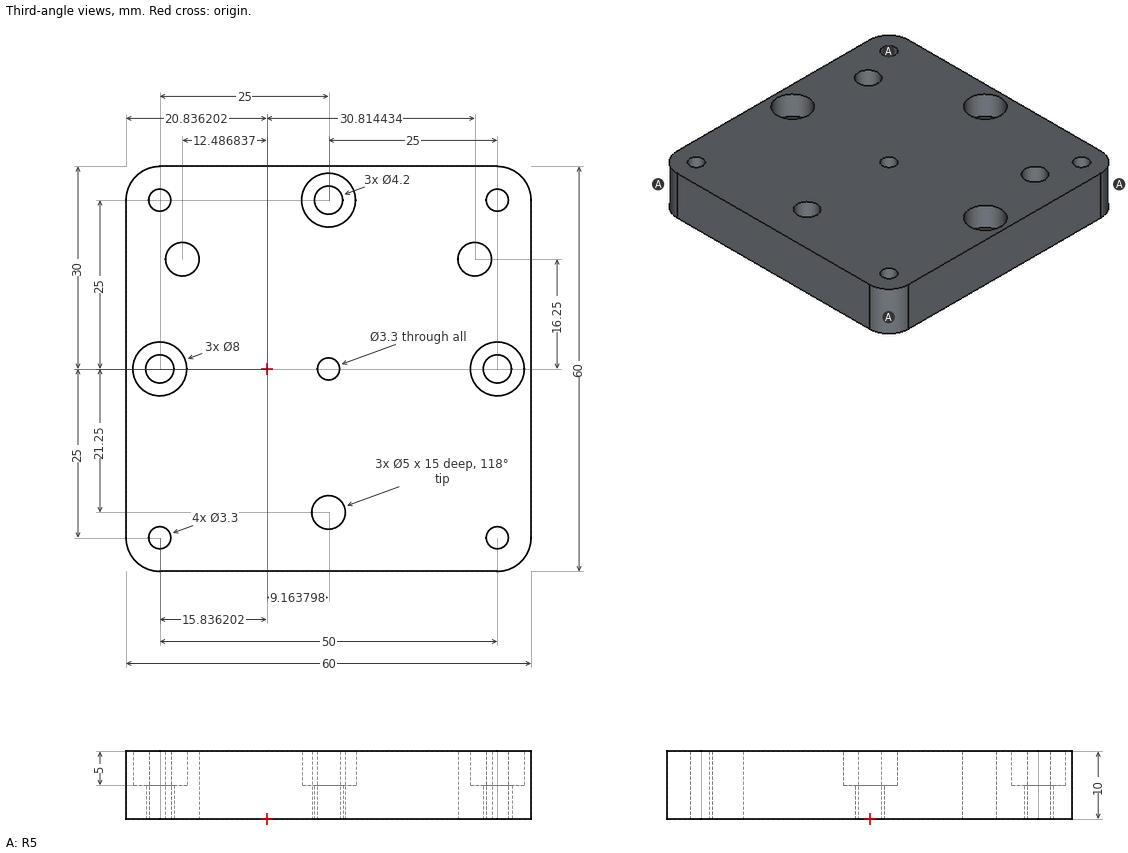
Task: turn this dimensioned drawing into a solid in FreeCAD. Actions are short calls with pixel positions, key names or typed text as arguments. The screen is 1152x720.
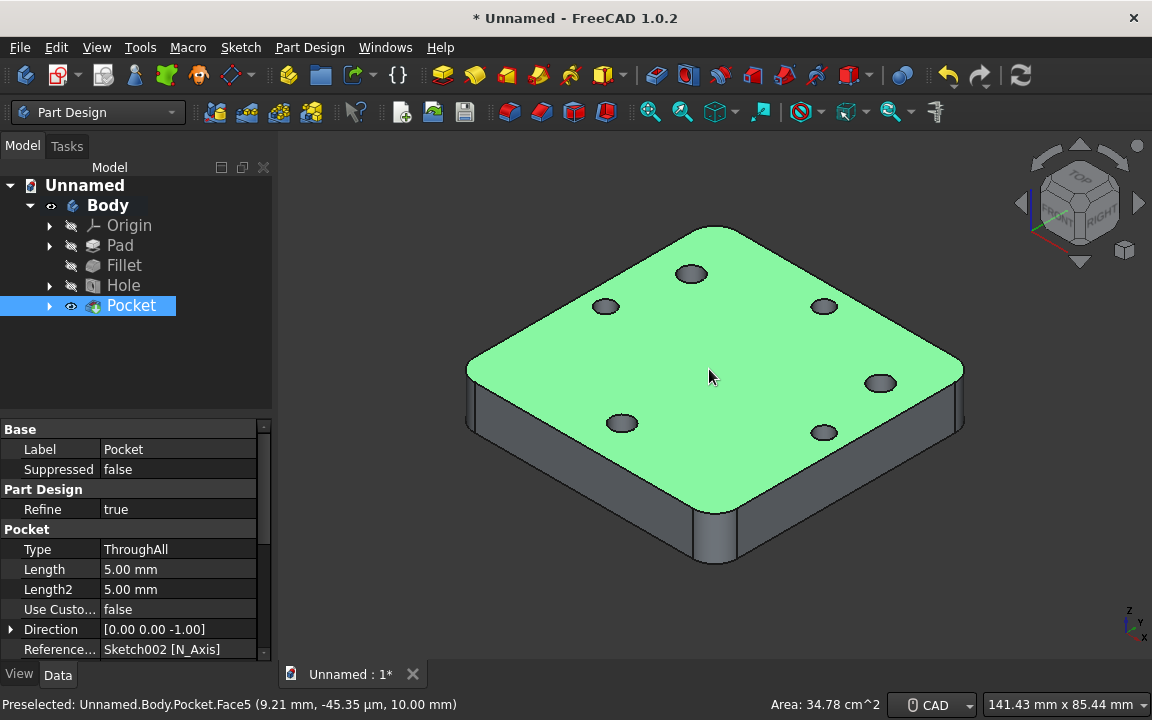
click(58, 76)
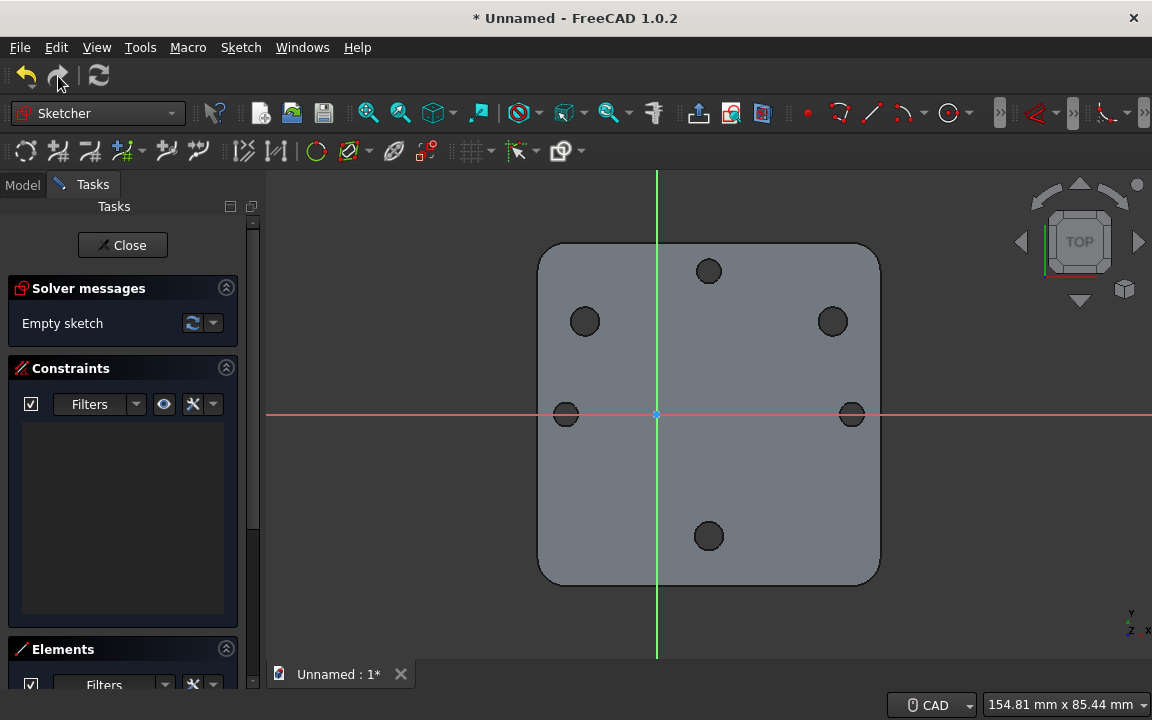
scroll(848, 198, up, 2)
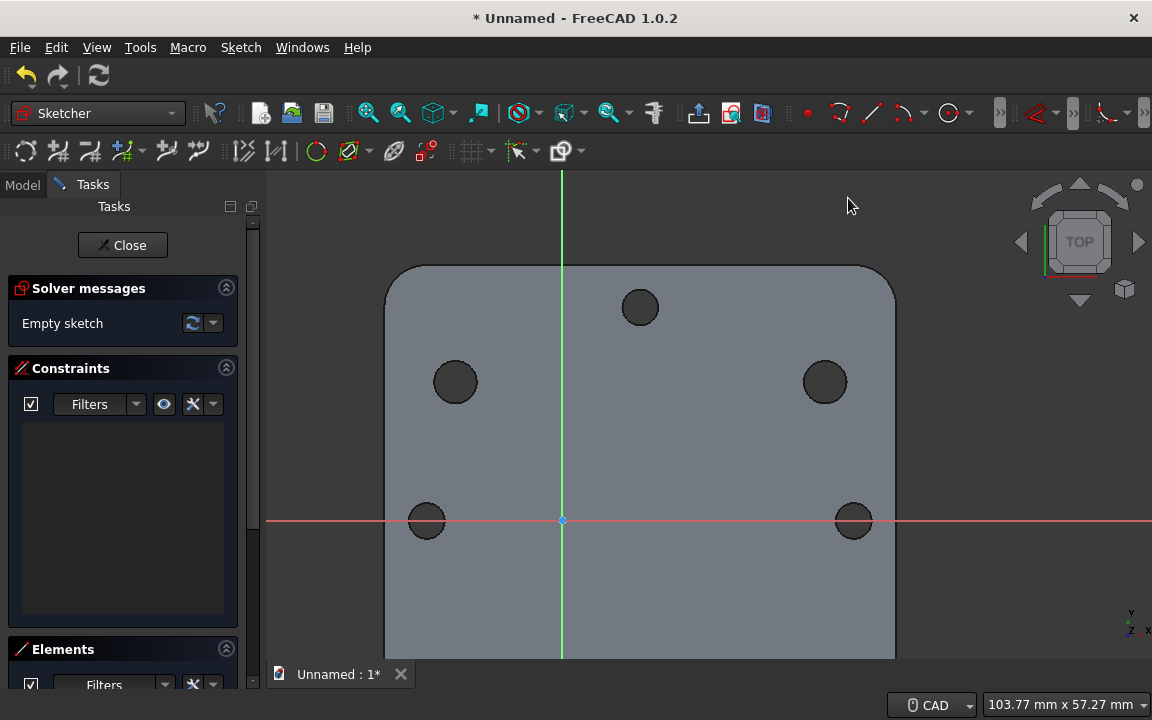
click(950, 114)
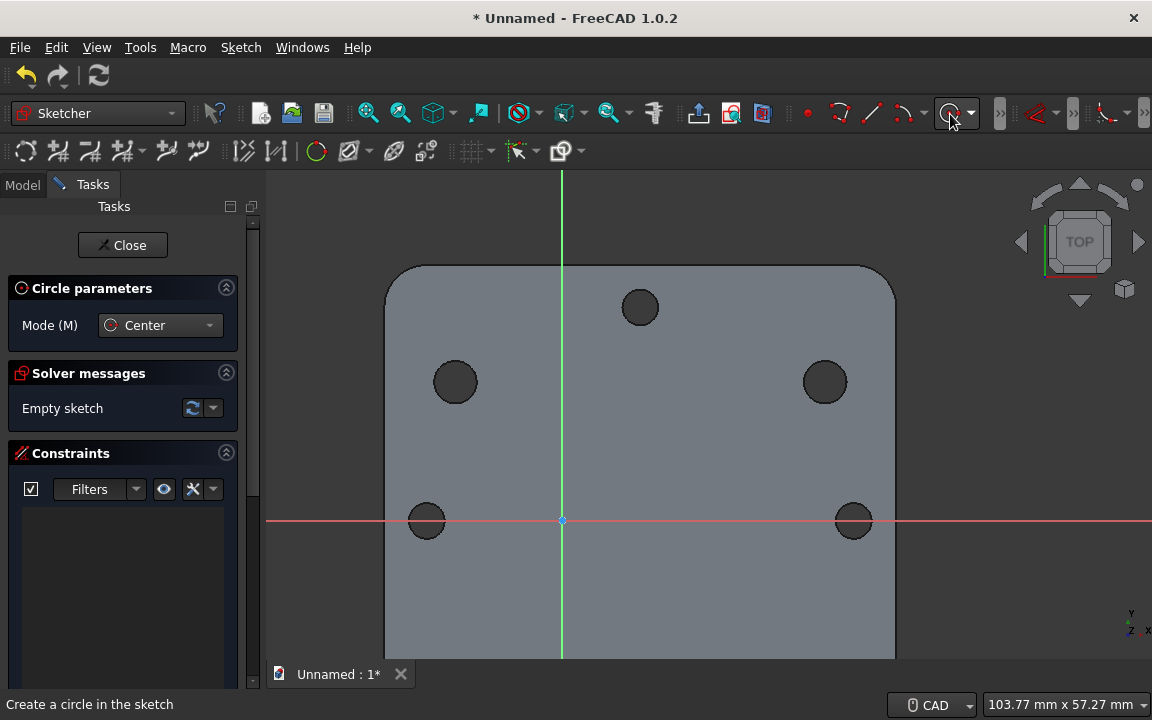
click(427, 521)
move(451, 497)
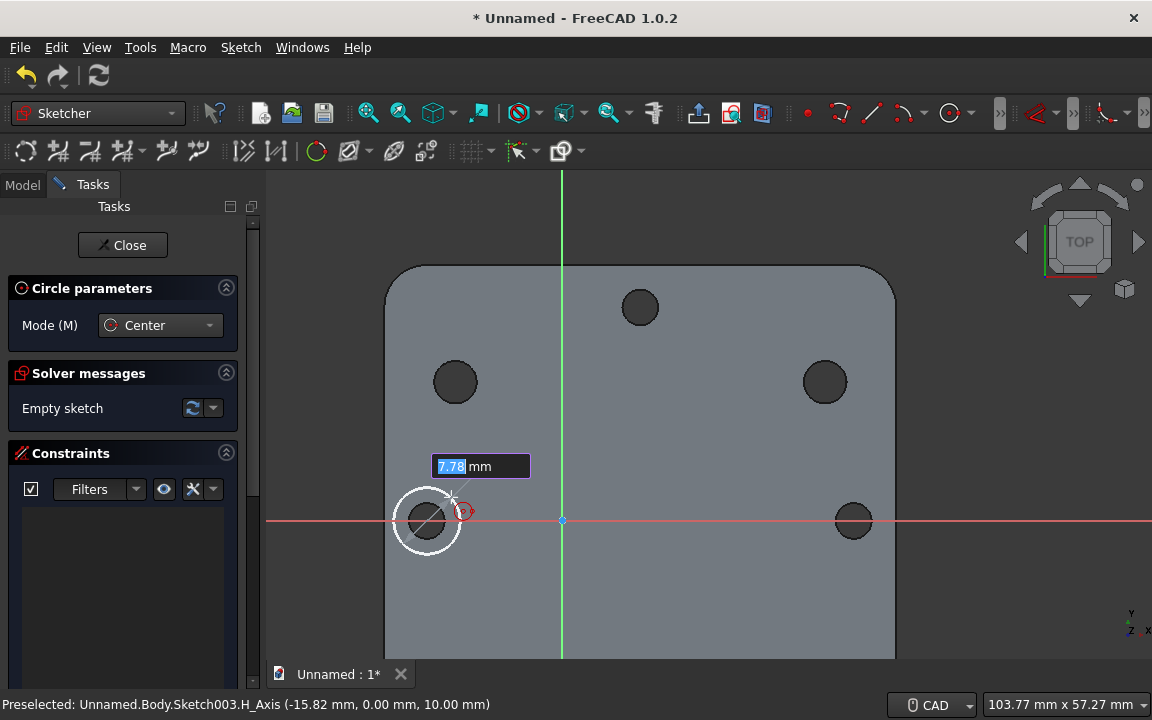
text(8)
key(Return)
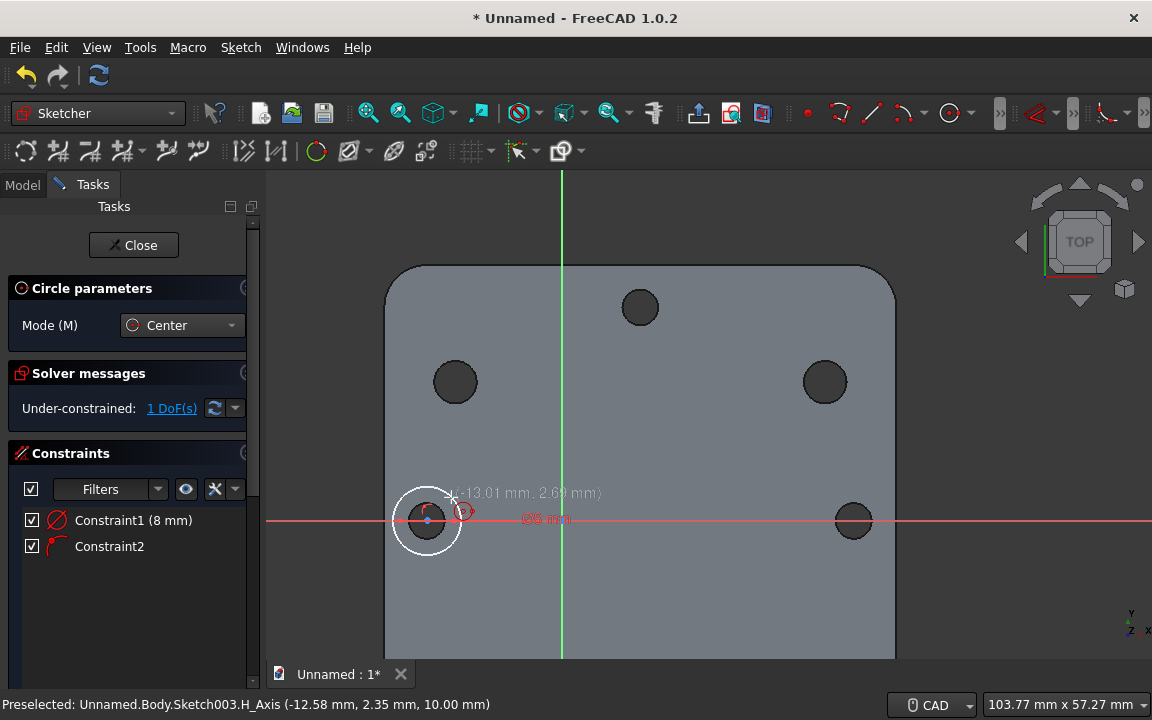
click(640, 307)
move(664, 283)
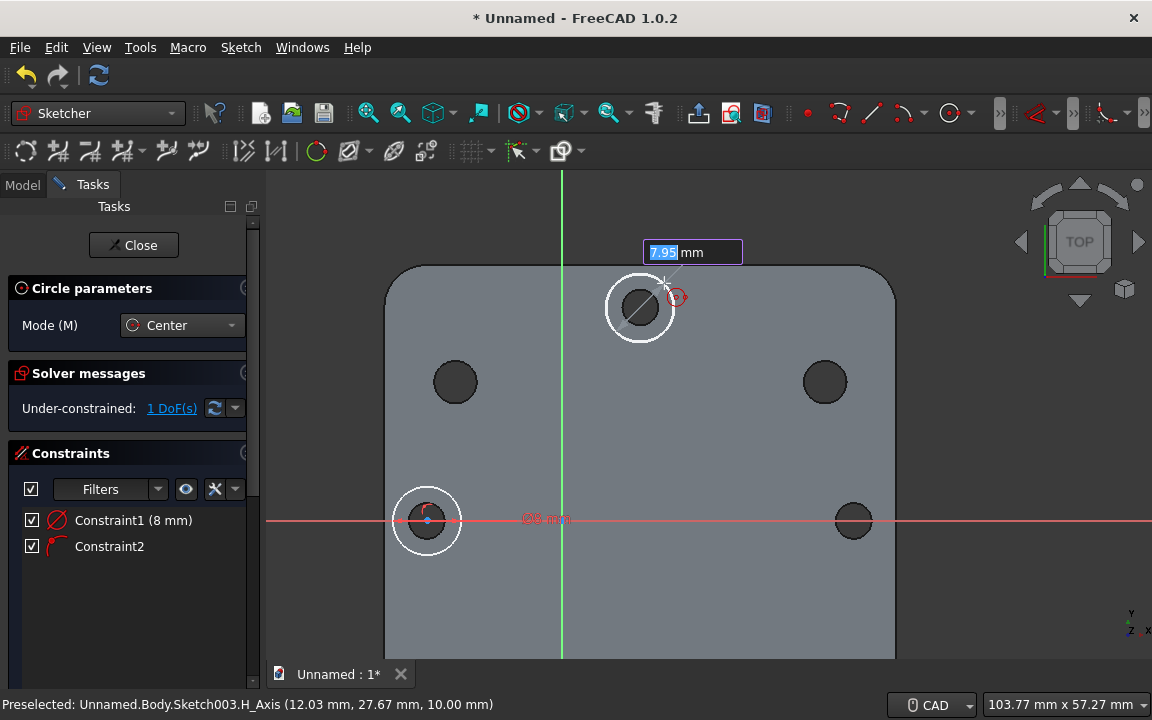
text(8)
key(Return)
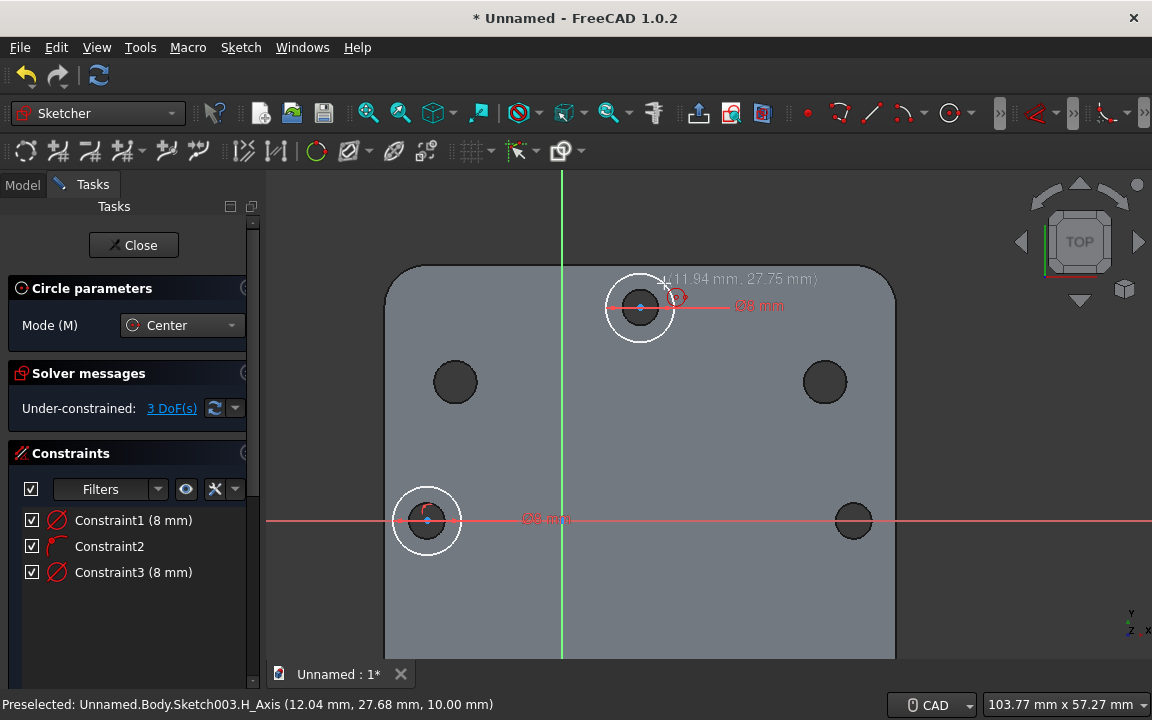
click(854, 521)
move(878, 497)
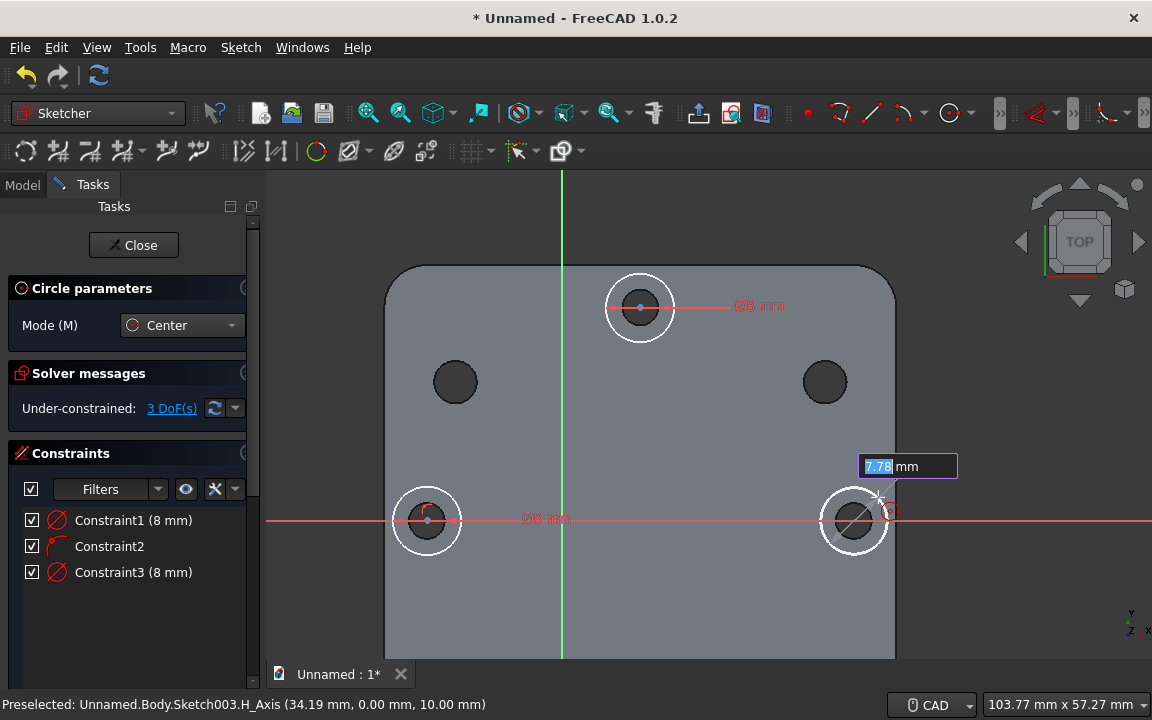
text(8)
key(Return)
key(Escape)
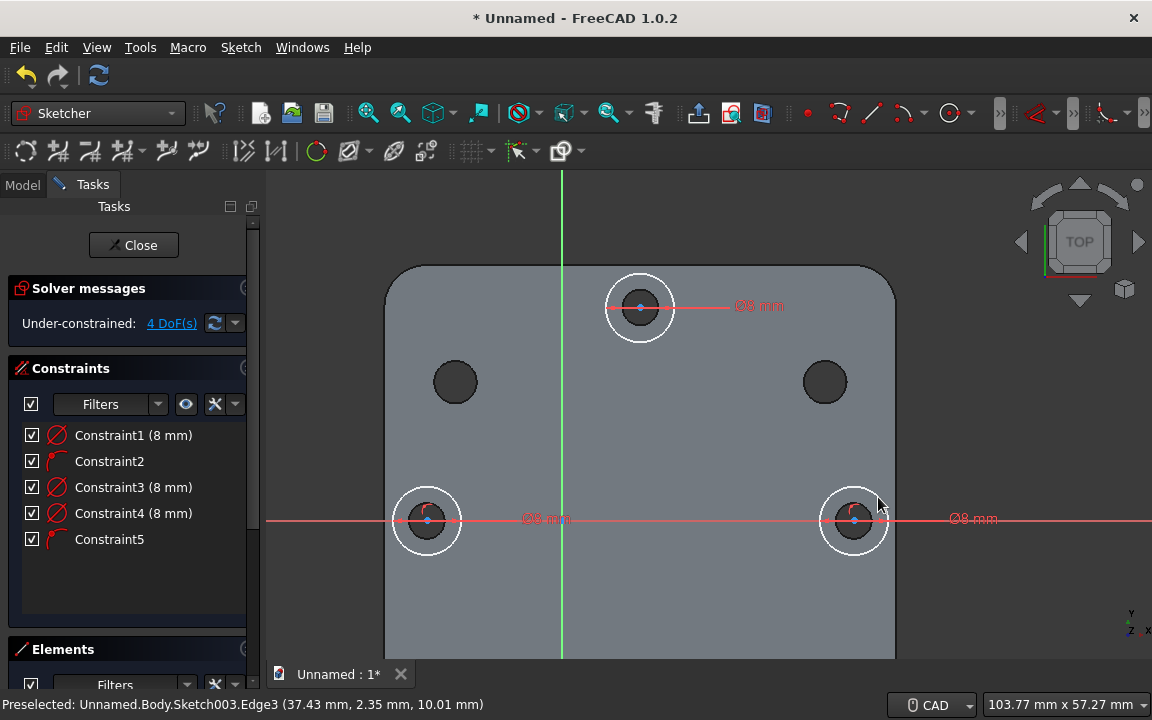
click(1036, 114)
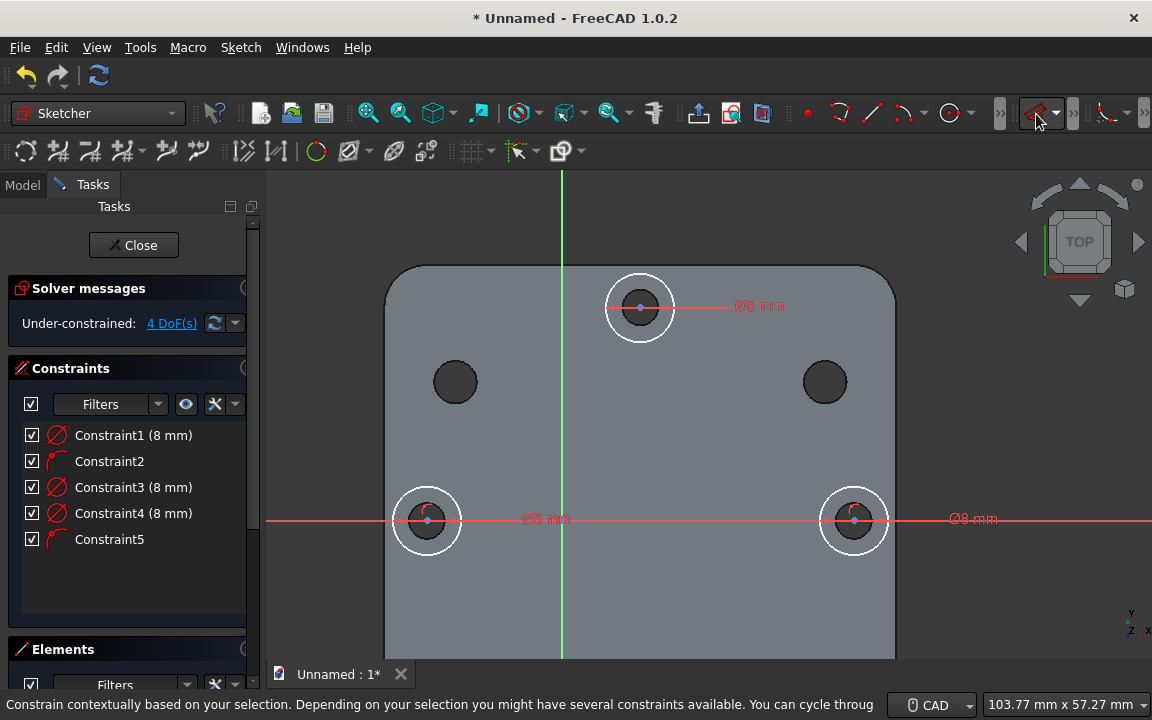
click(640, 308)
click(528, 414)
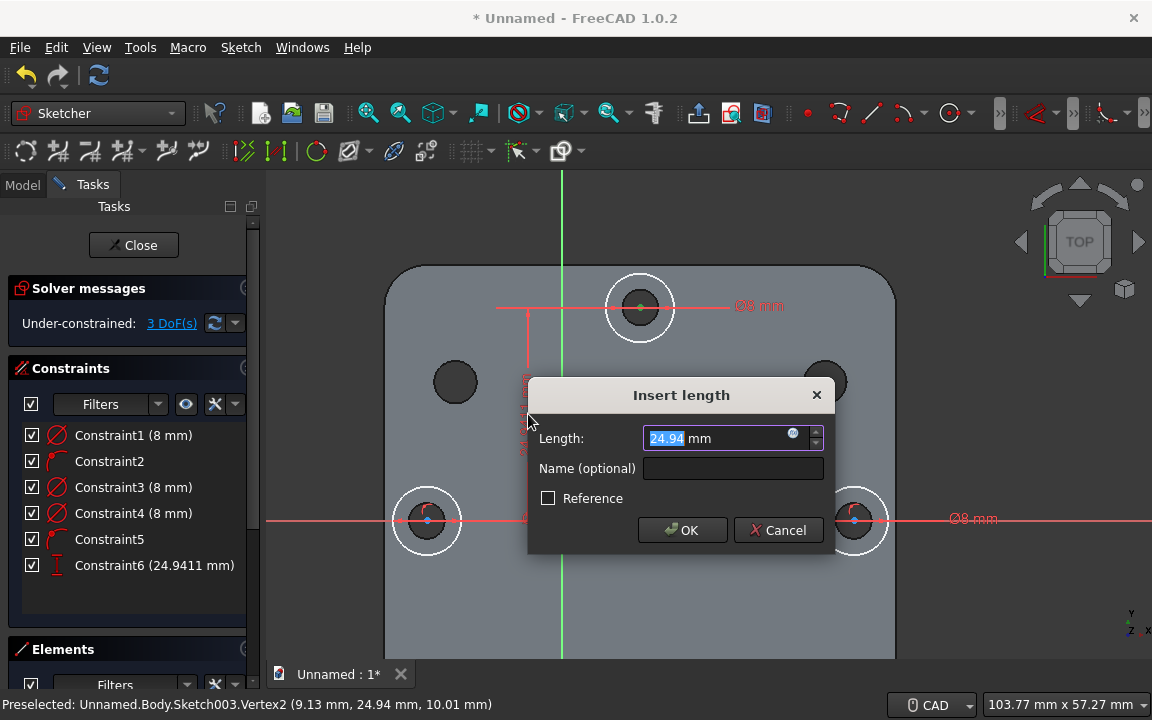
text(25)
key(Return)